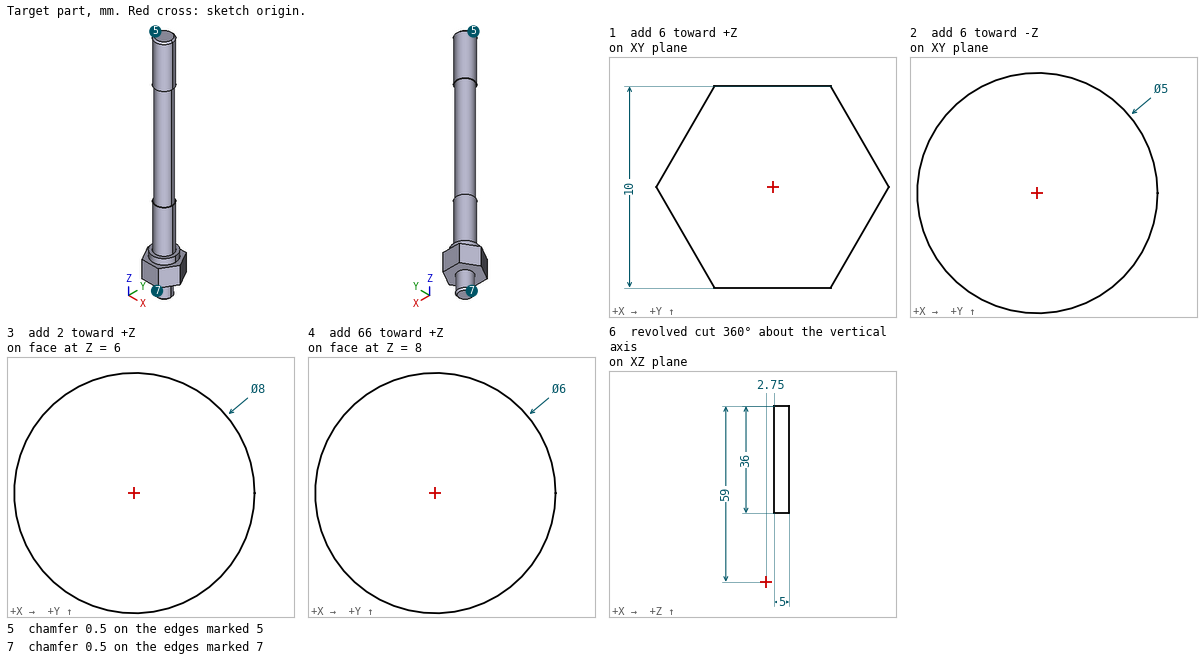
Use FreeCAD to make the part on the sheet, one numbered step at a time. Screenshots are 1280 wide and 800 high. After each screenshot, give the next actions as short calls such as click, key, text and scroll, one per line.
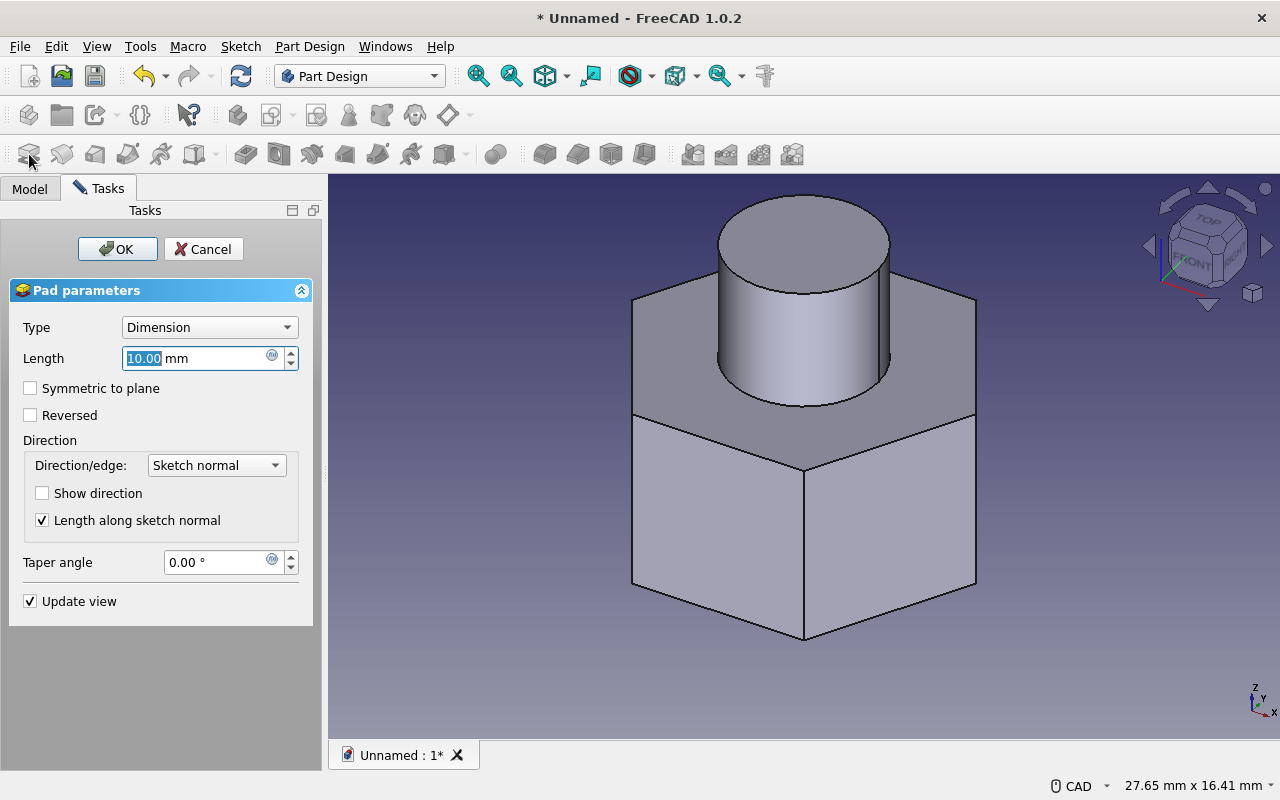
text(6)
key(Tab)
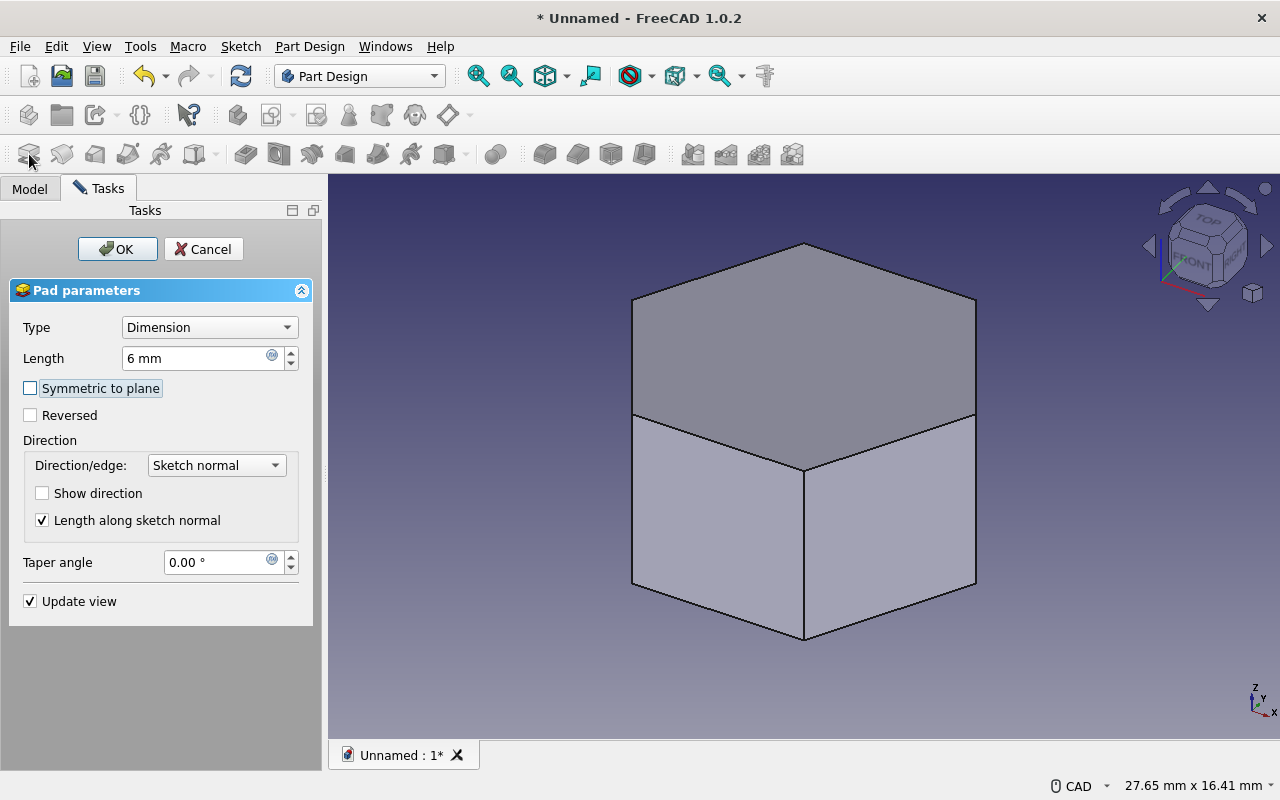
click(31, 415)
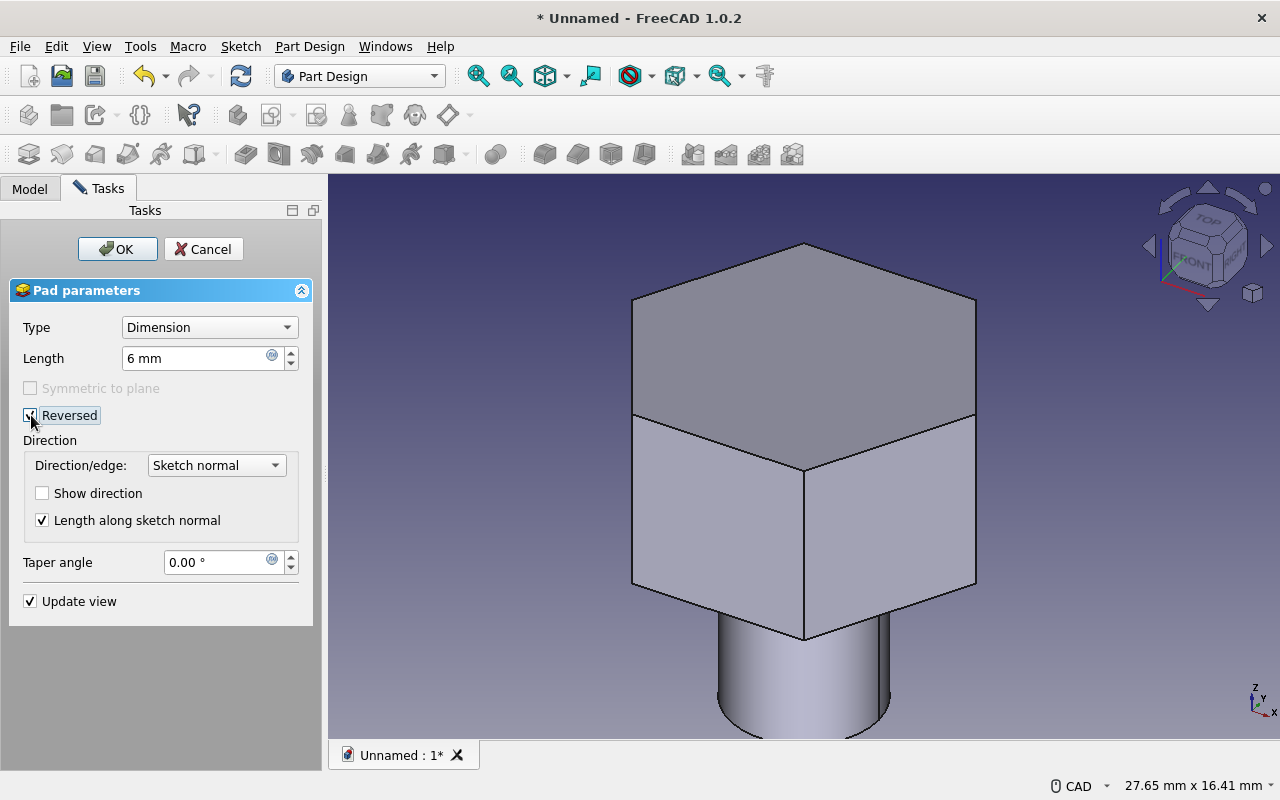
click(118, 249)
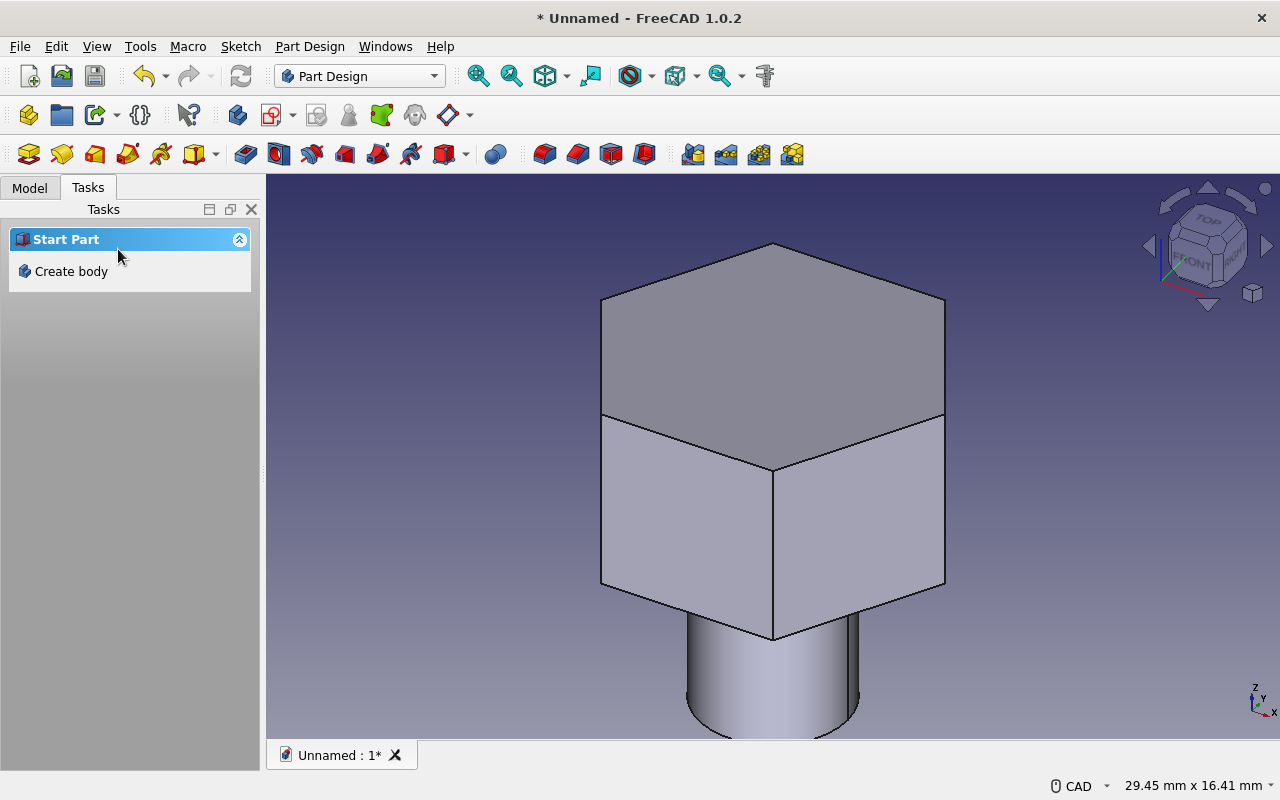
click(479, 76)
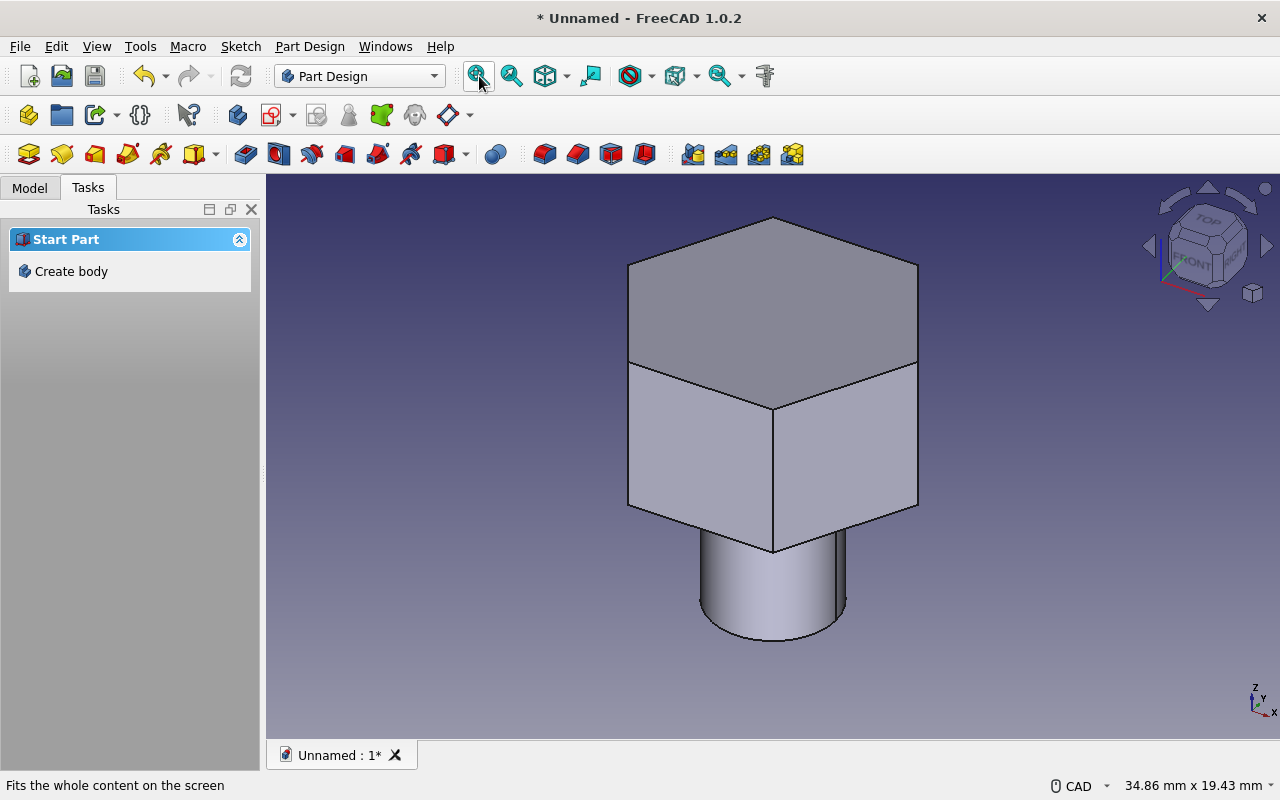
click(773, 313)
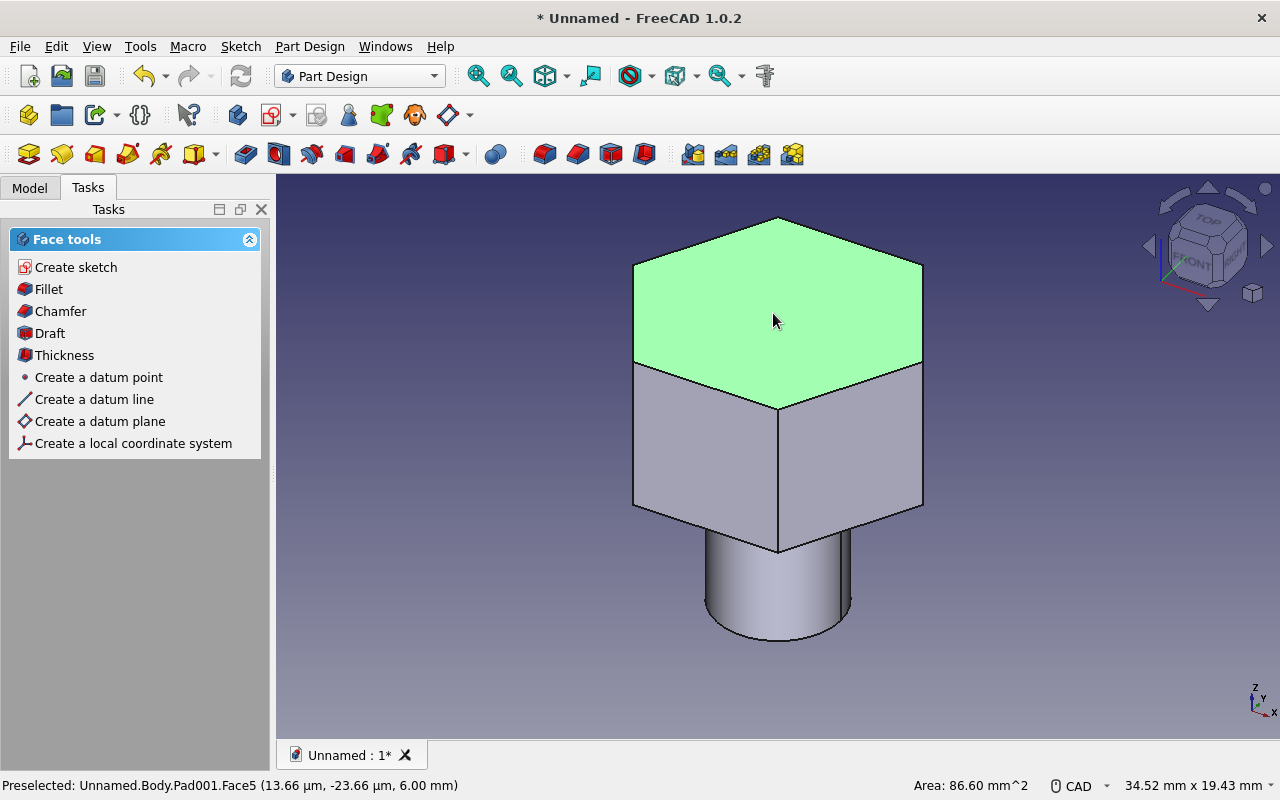
click(270, 116)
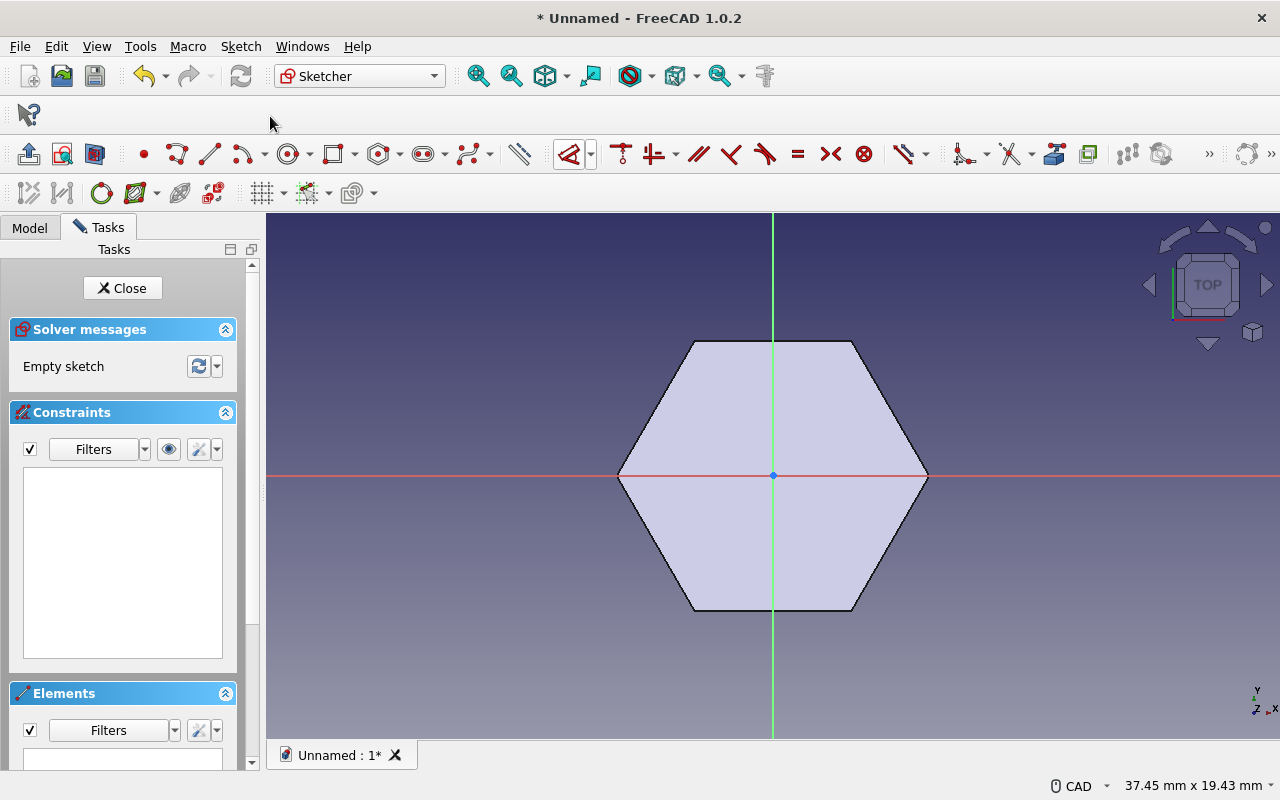
scroll(912, 476, up, 2)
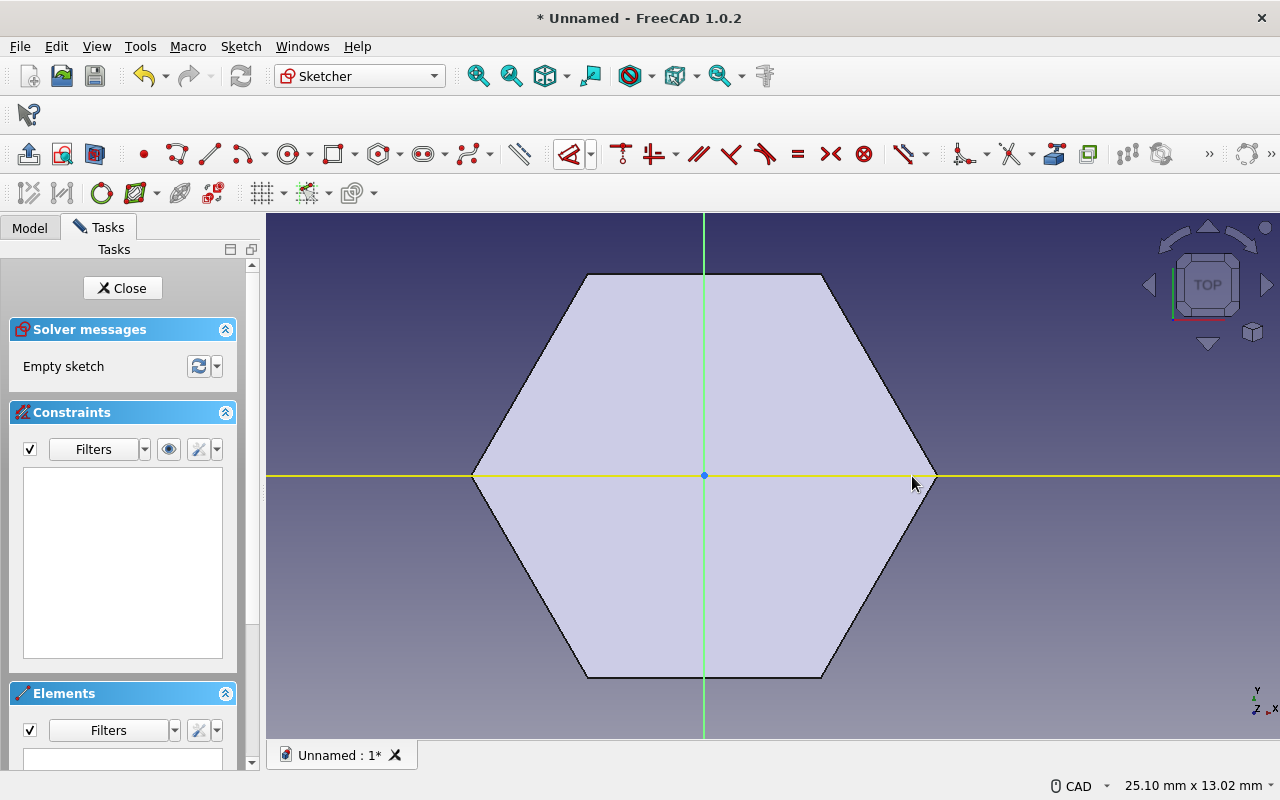
click(288, 154)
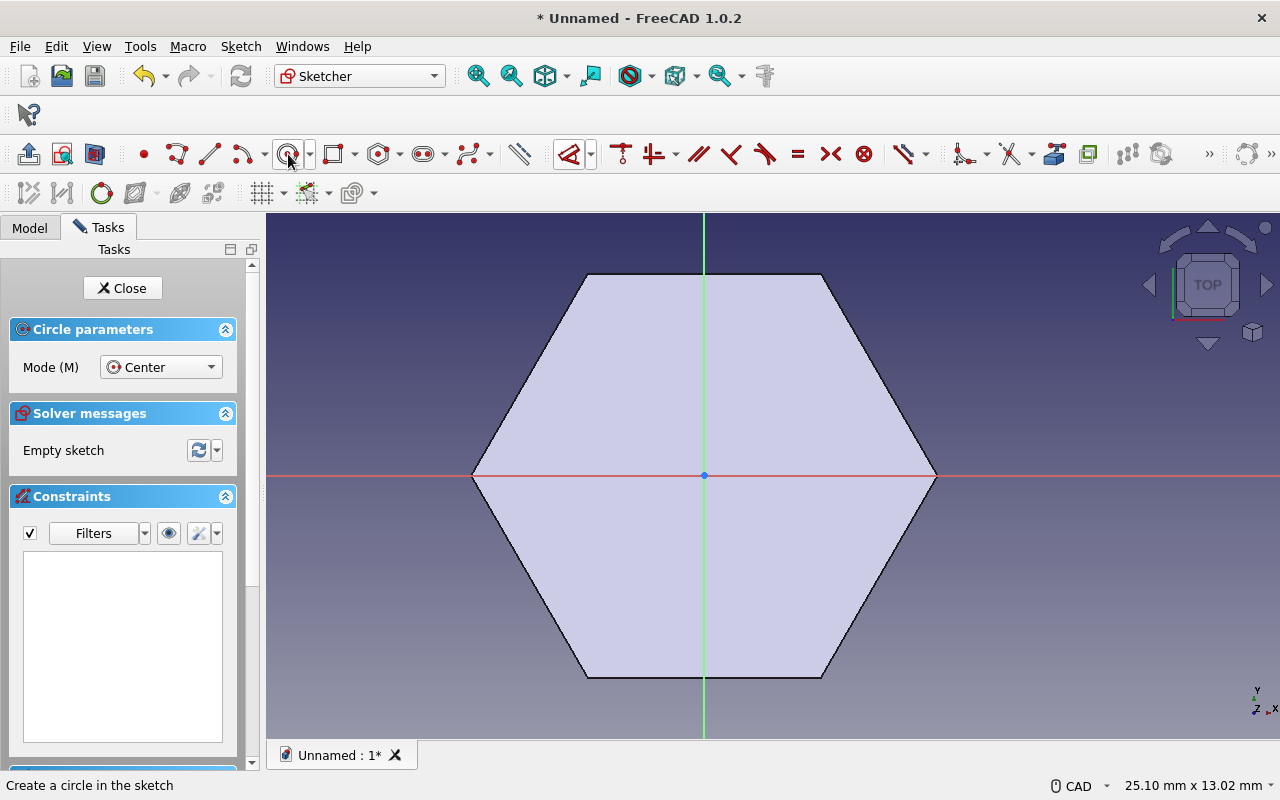
click(704, 476)
click(819, 361)
key(Escape)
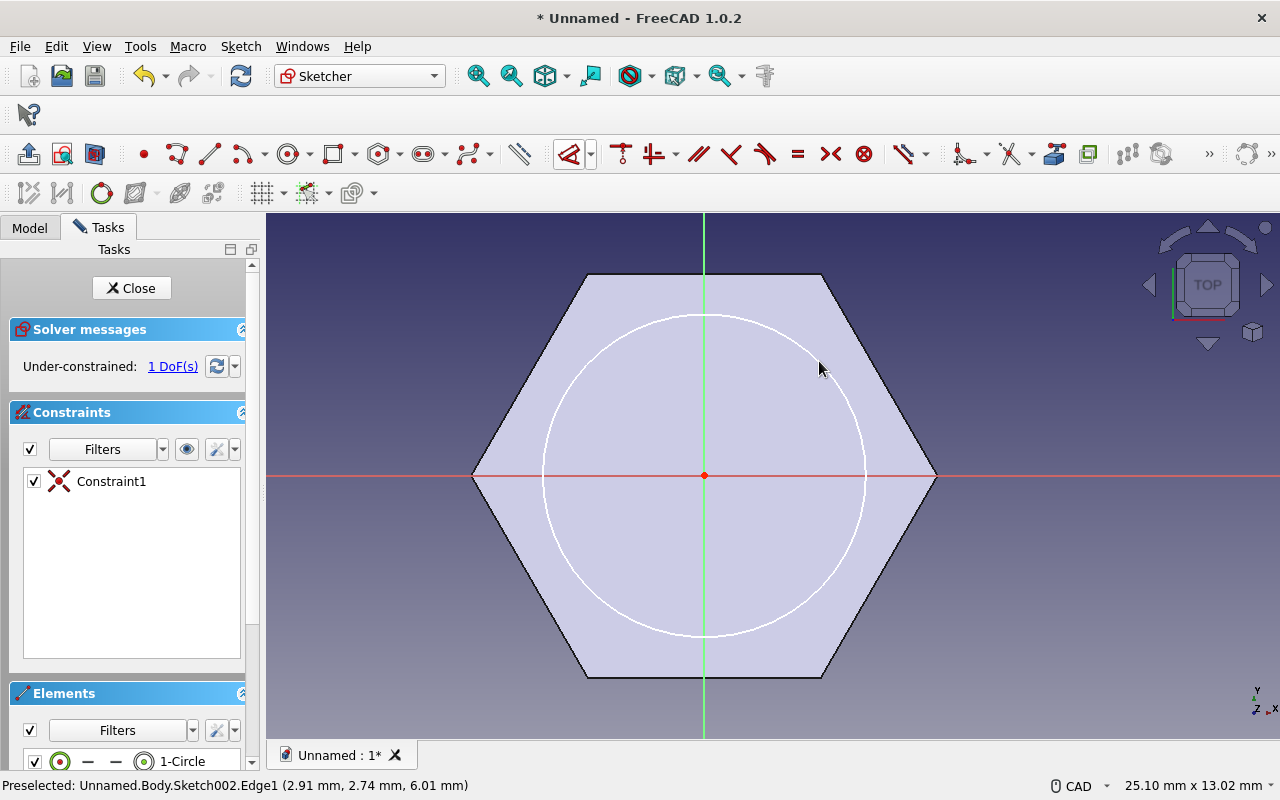
click(818, 361)